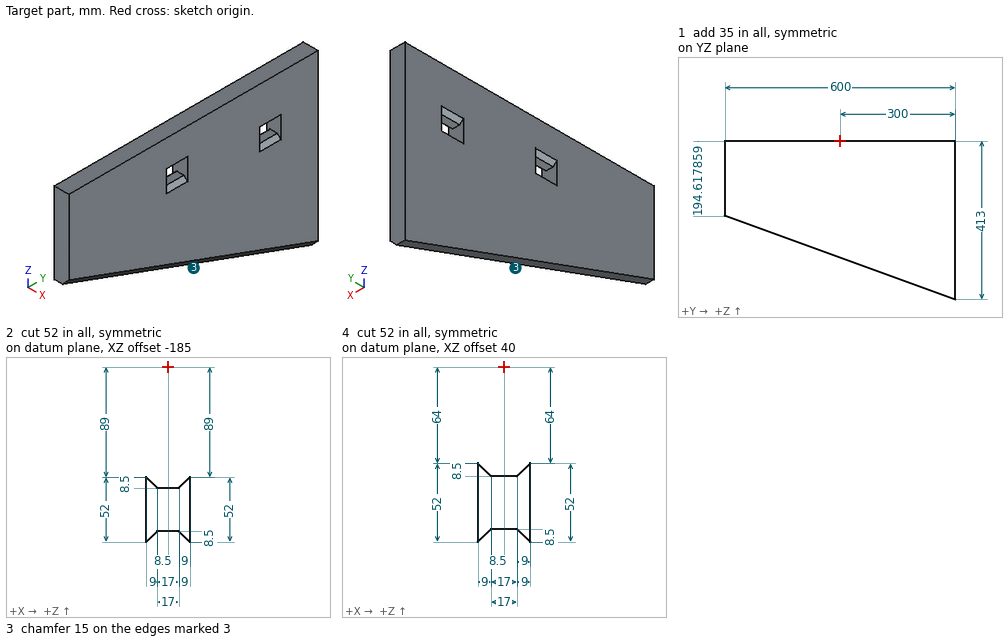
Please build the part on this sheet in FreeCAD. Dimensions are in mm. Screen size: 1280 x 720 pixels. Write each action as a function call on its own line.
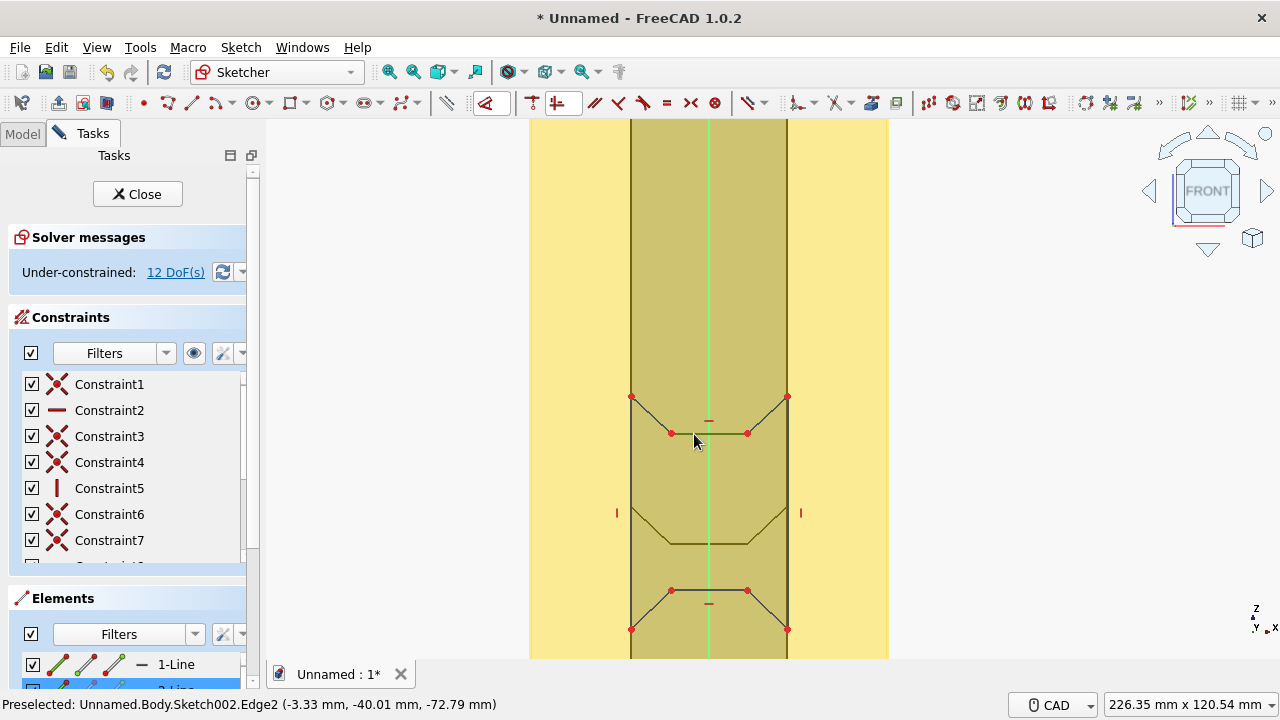
key(l)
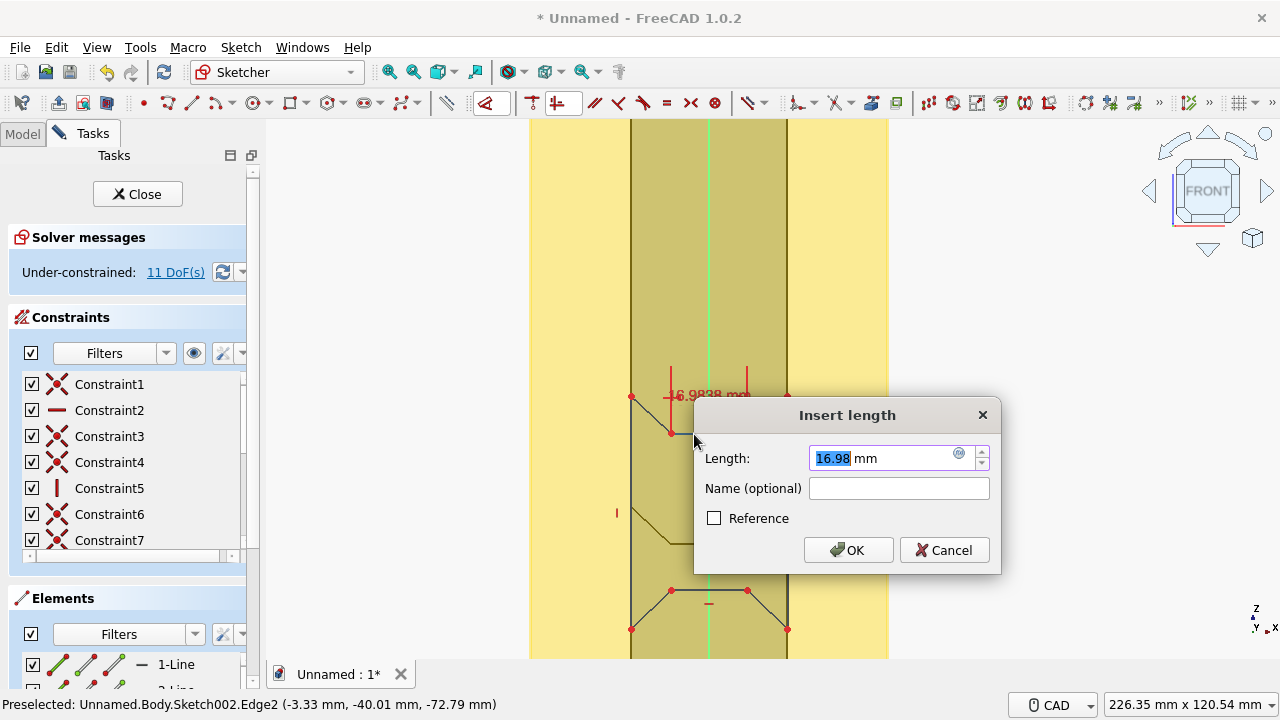
text(17)
key(Return)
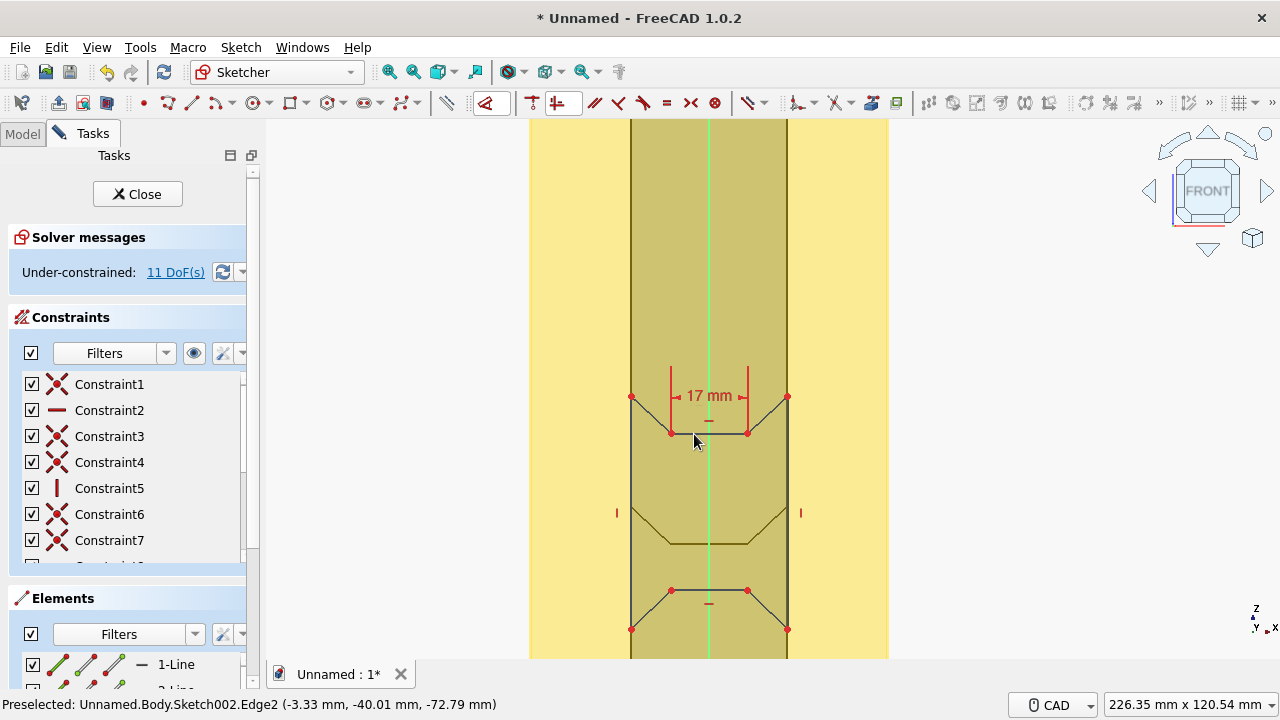
click(788, 466)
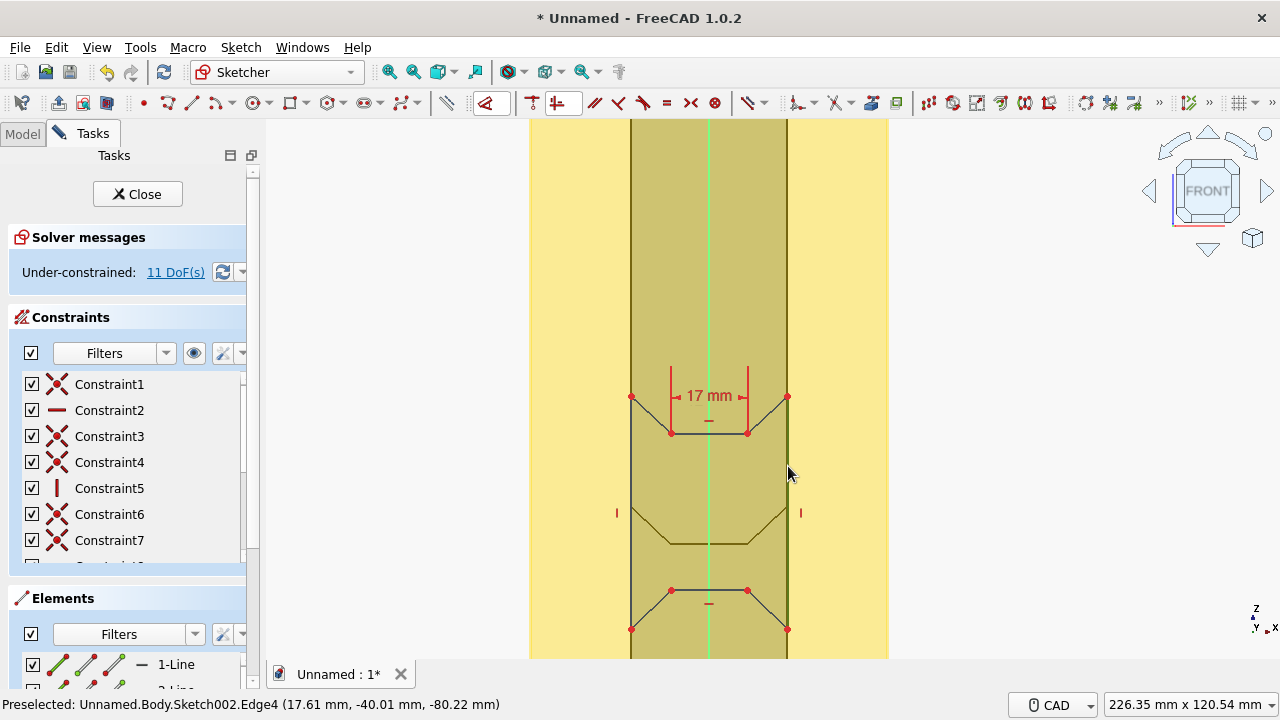
key(i)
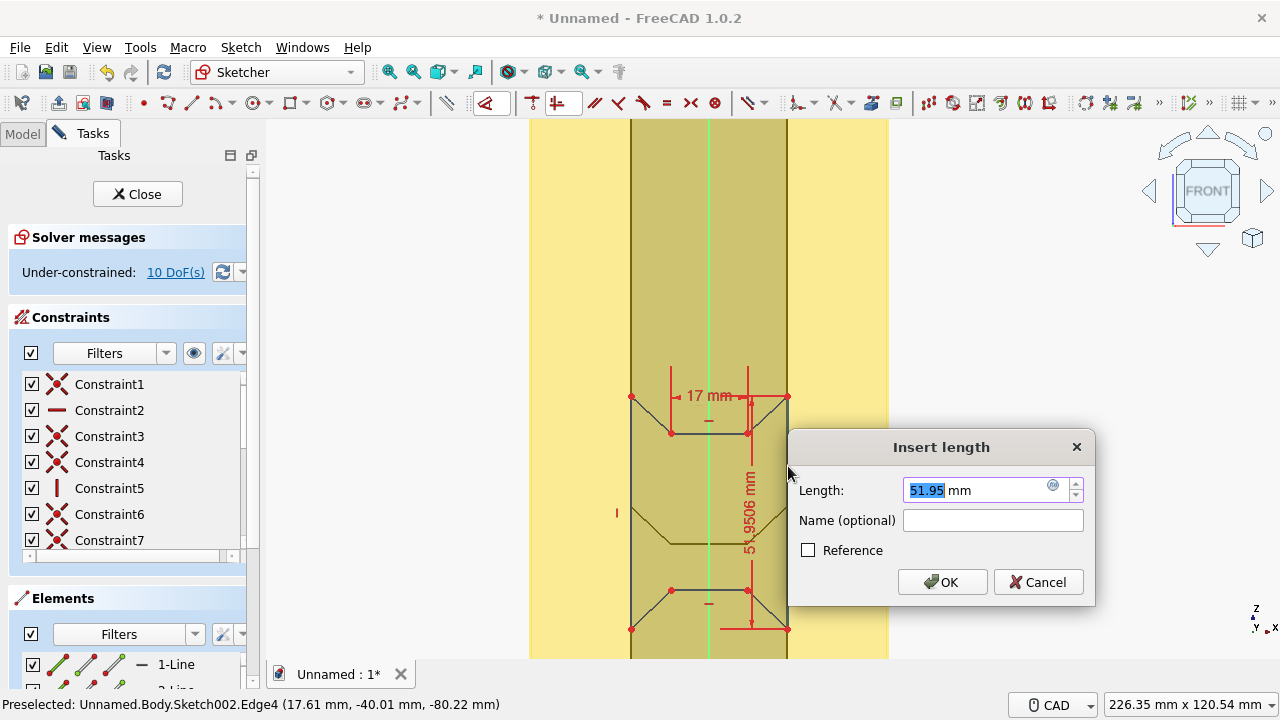
text(52)
key(Return)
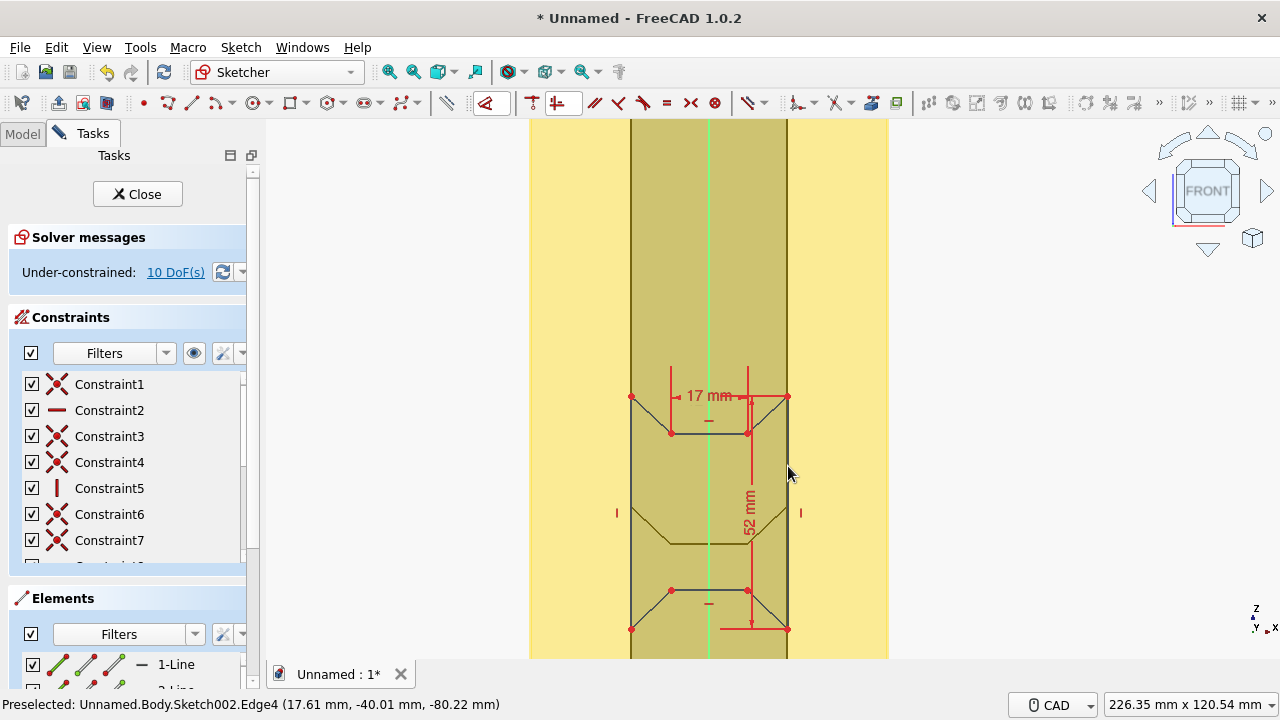
click(725, 590)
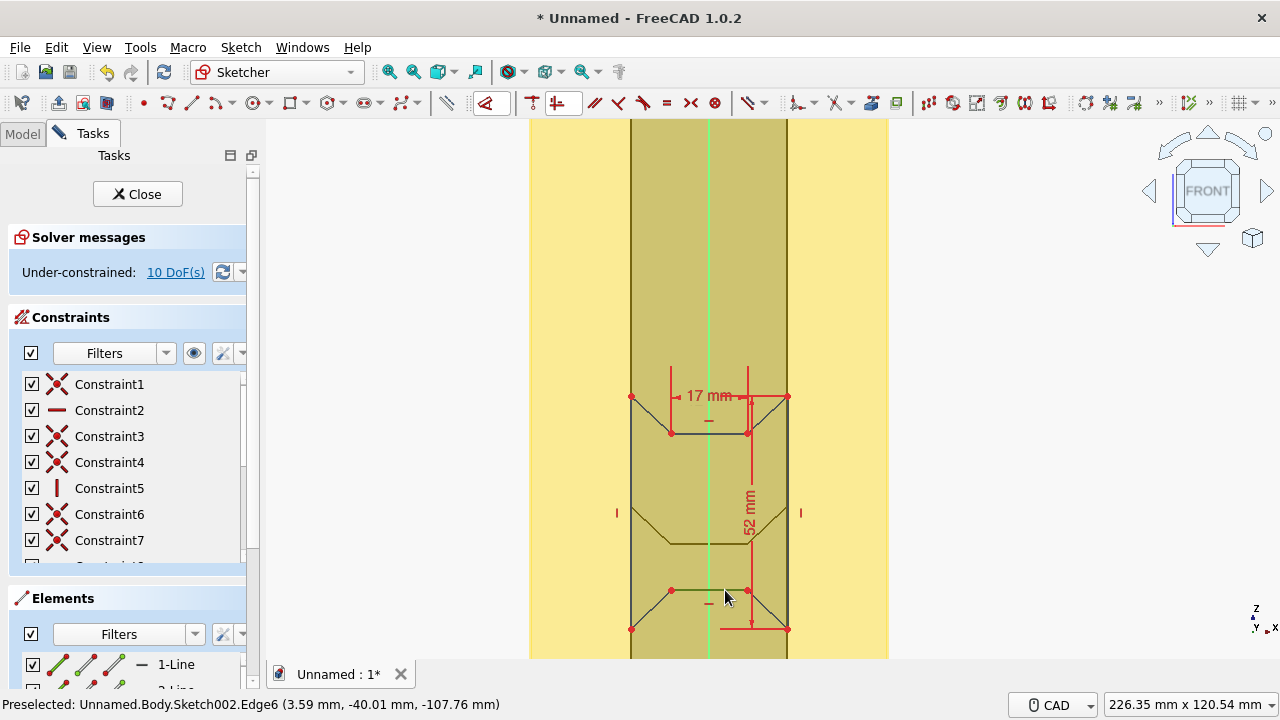
key(l)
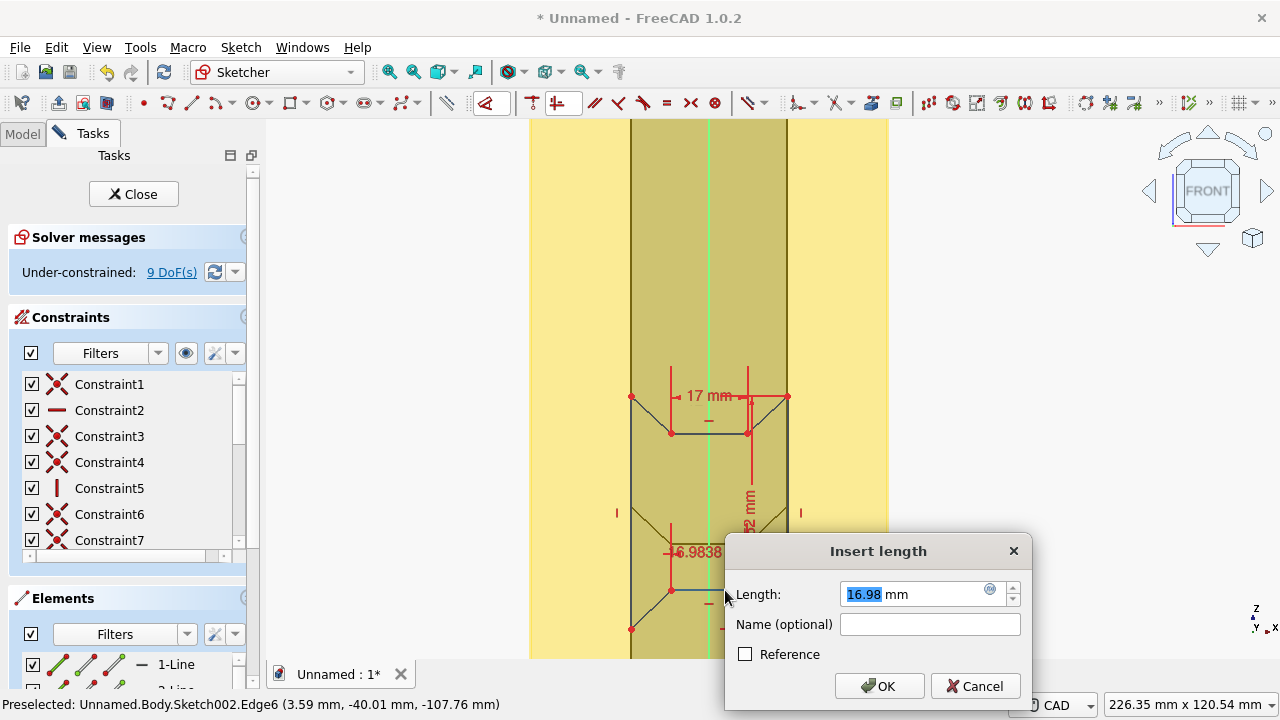
text(17)
key(Return)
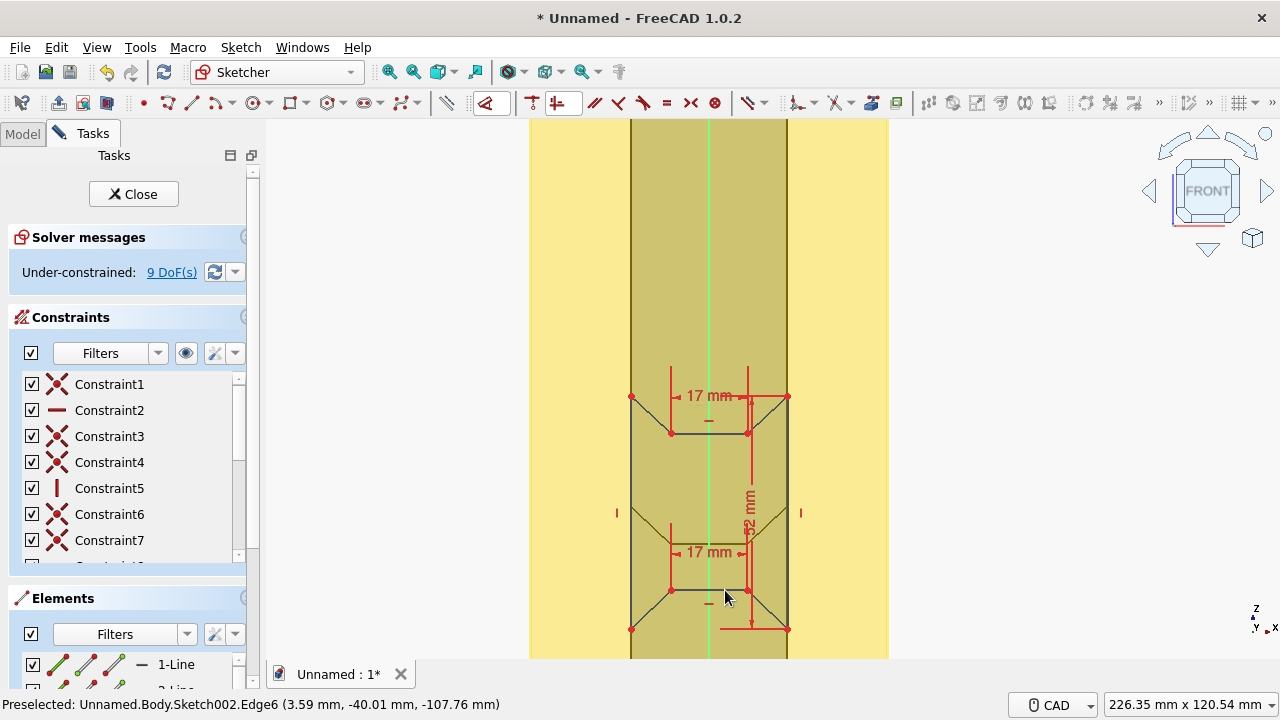
click(631, 559)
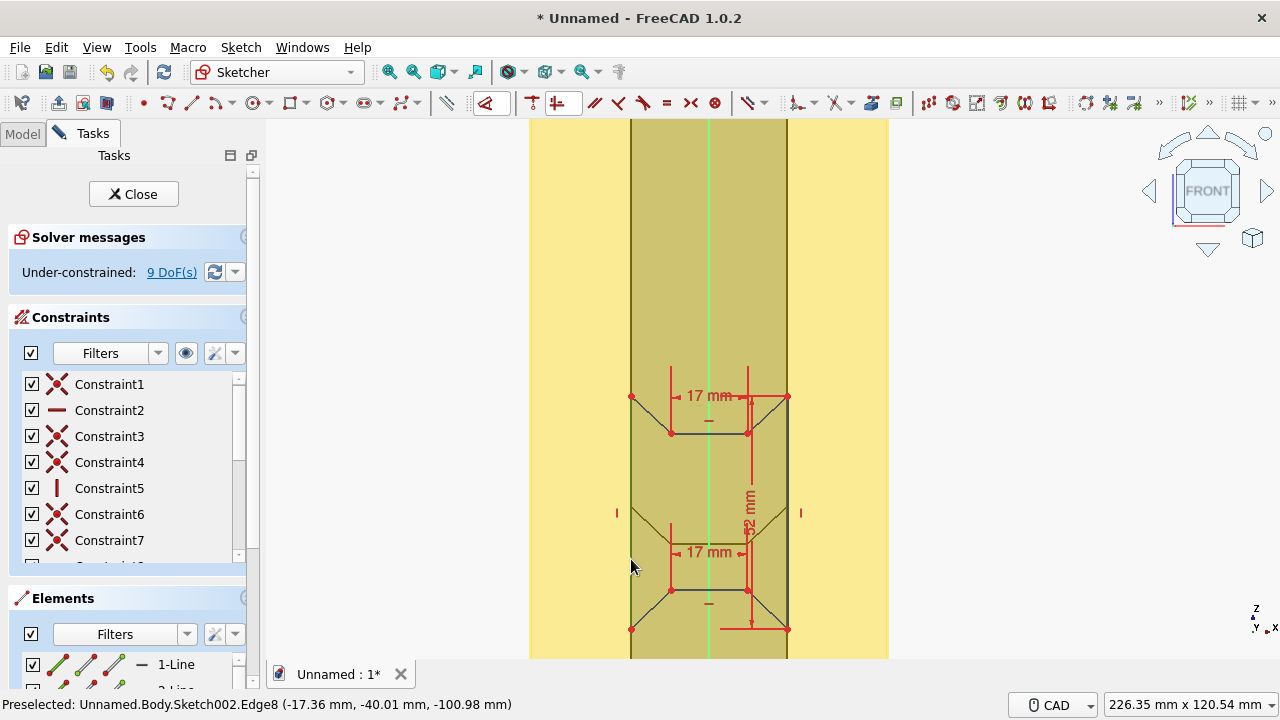
key(i)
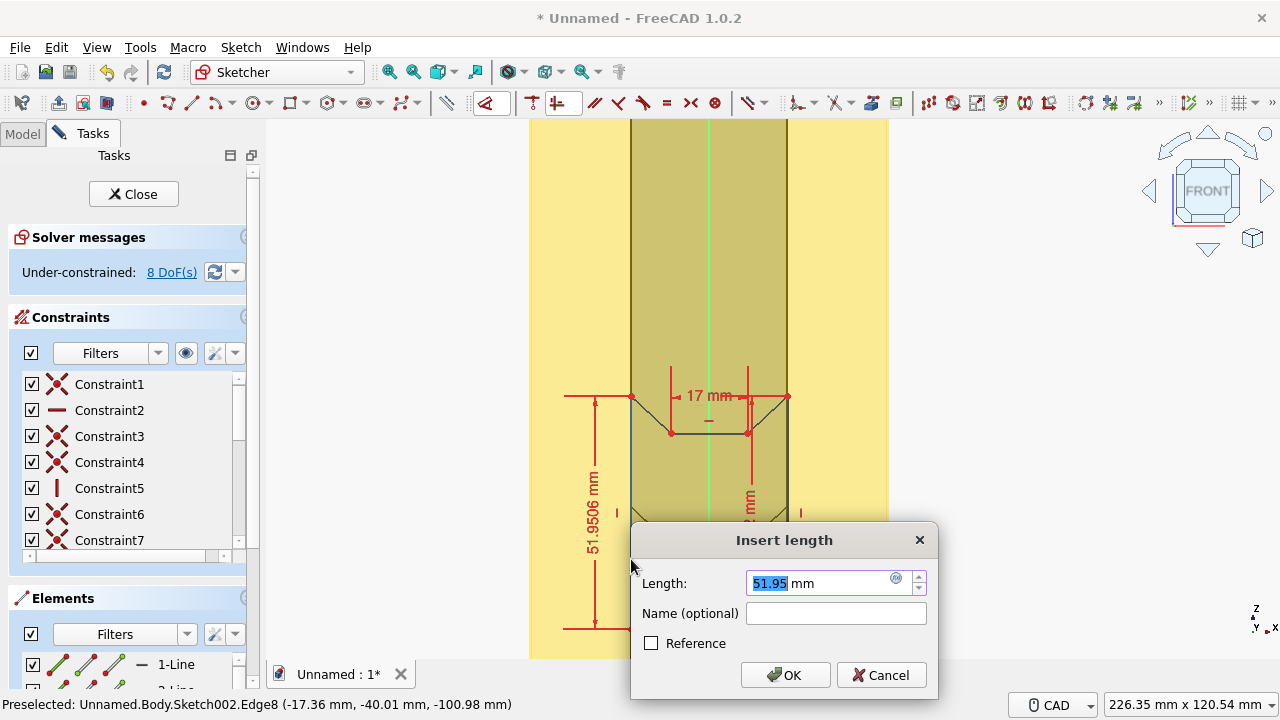
text(52)
key(Return)